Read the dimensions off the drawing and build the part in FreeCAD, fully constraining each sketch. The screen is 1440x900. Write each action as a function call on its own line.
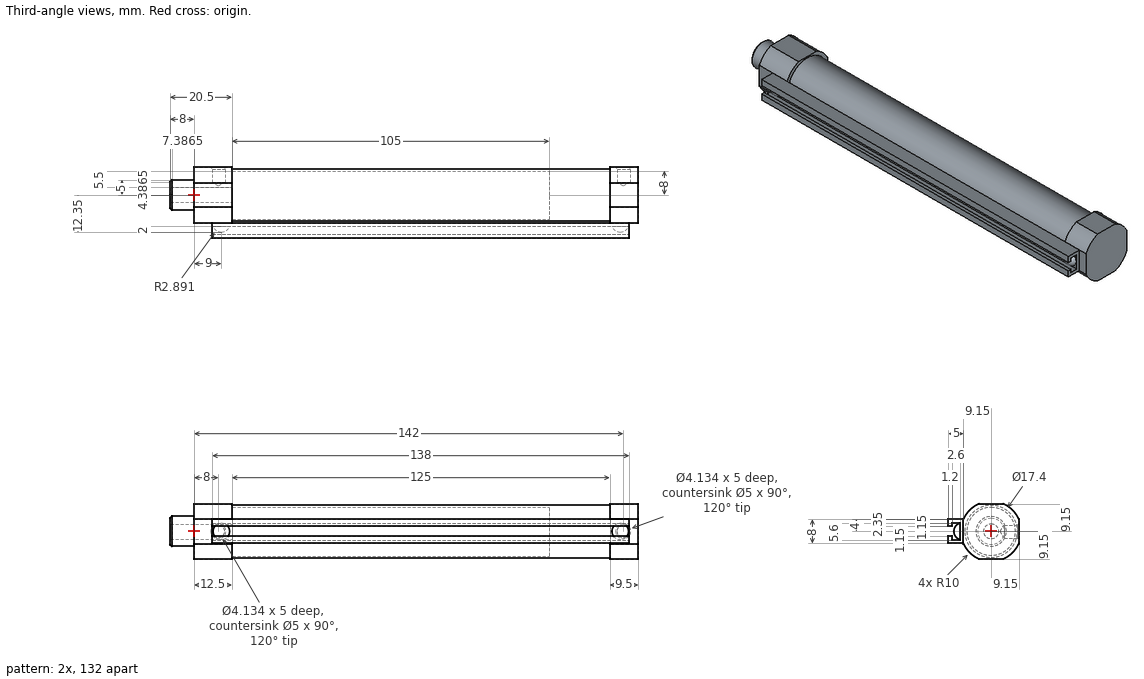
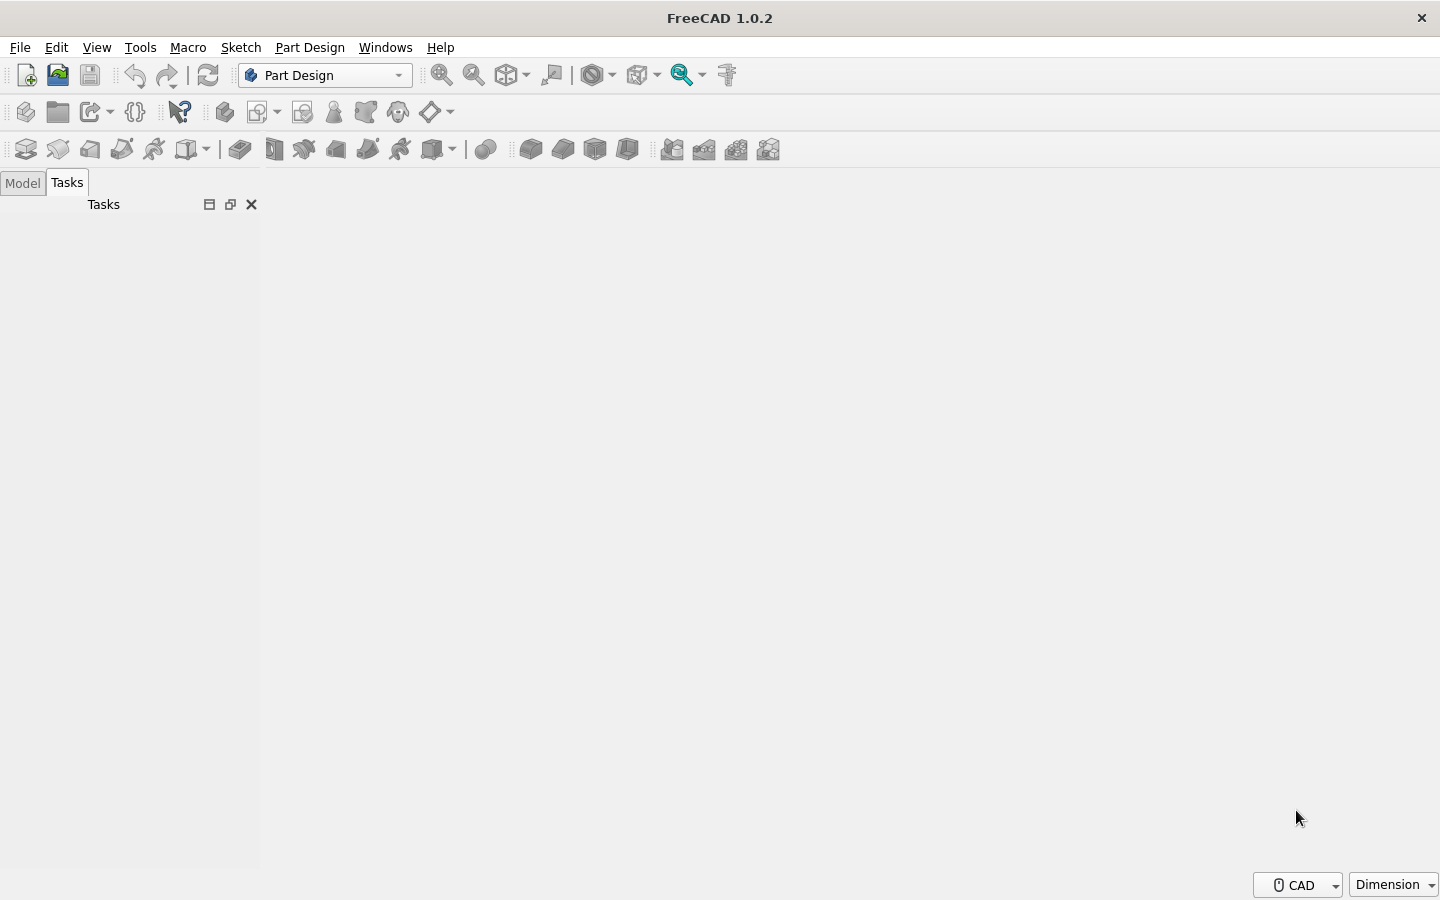
click(26, 76)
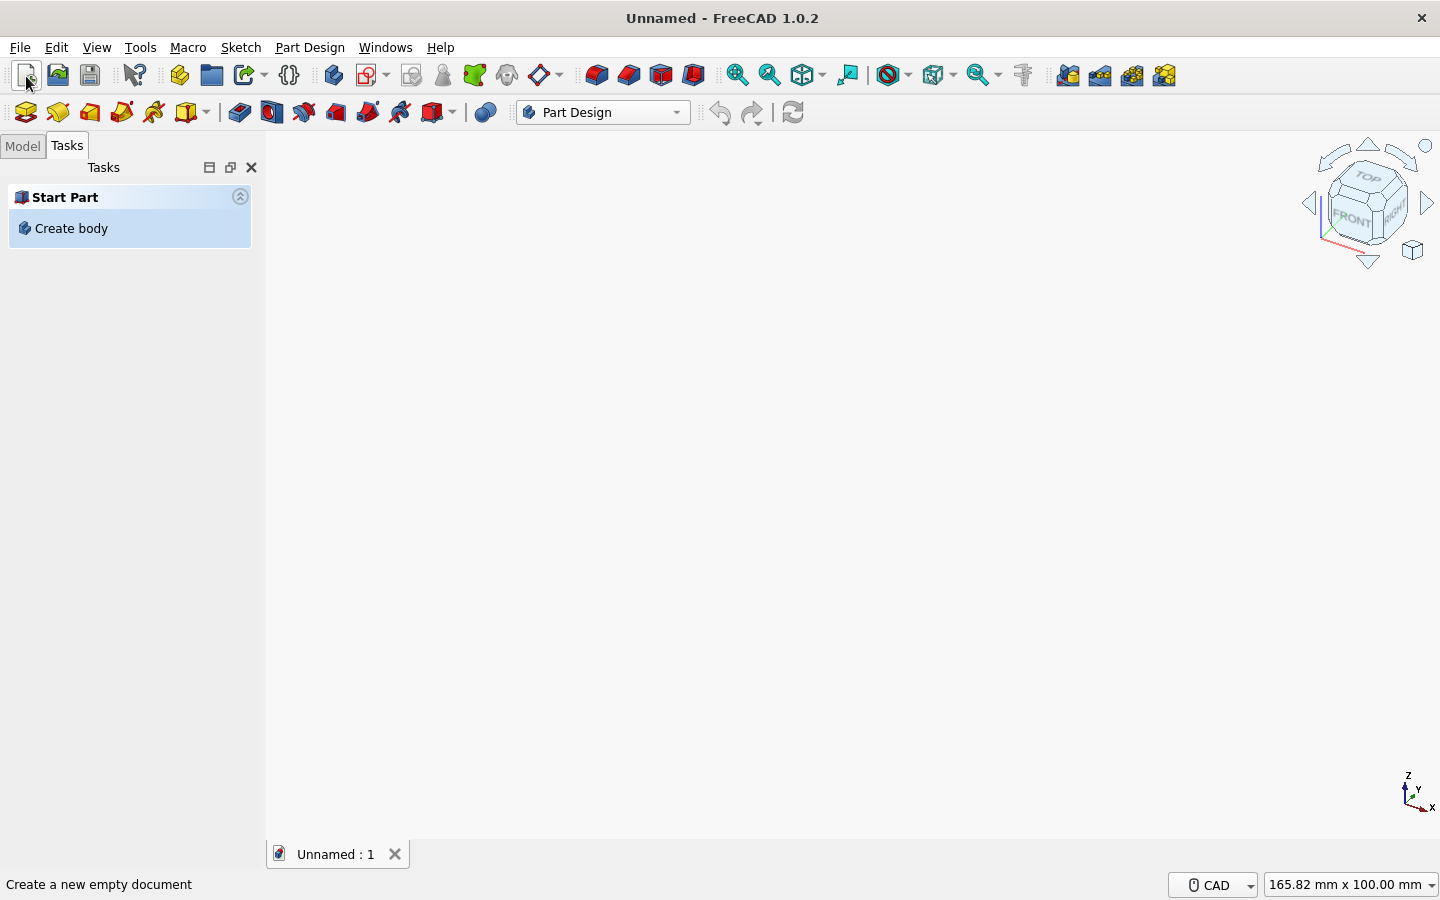
click(366, 76)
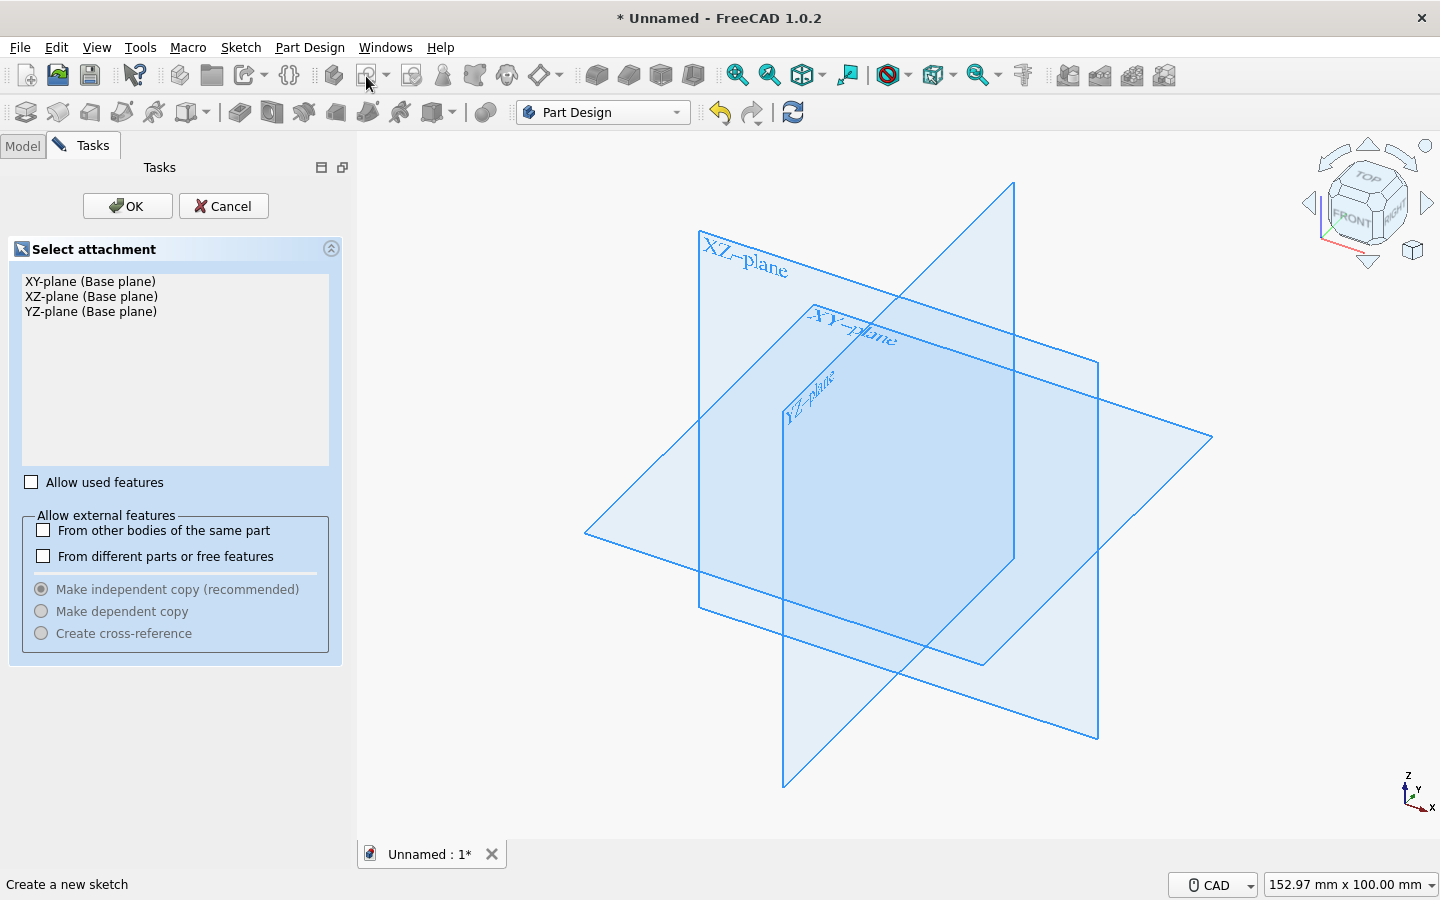
click(82, 282)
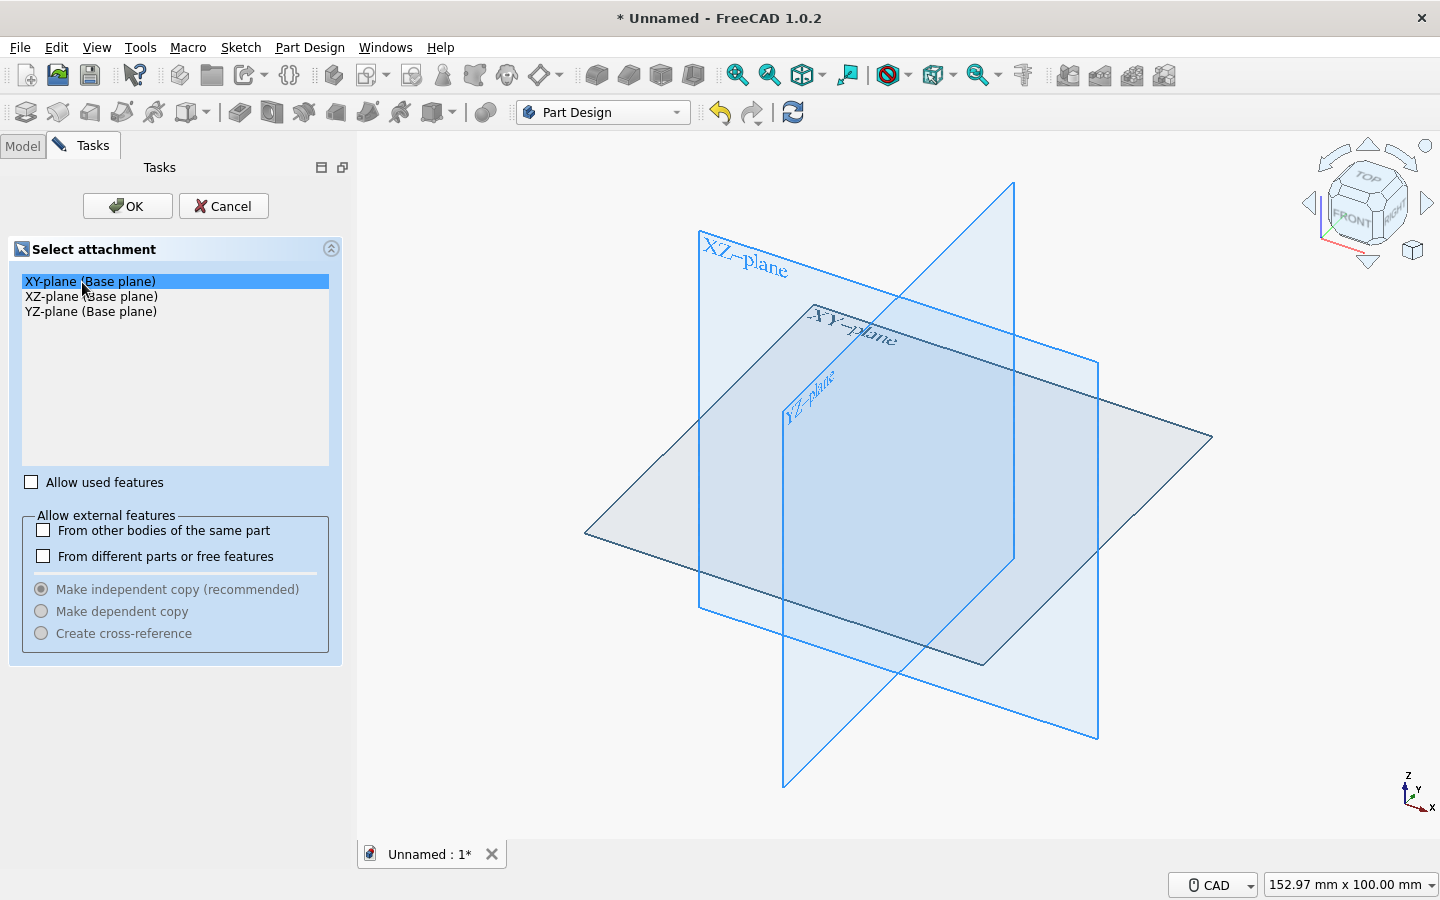
click(128, 206)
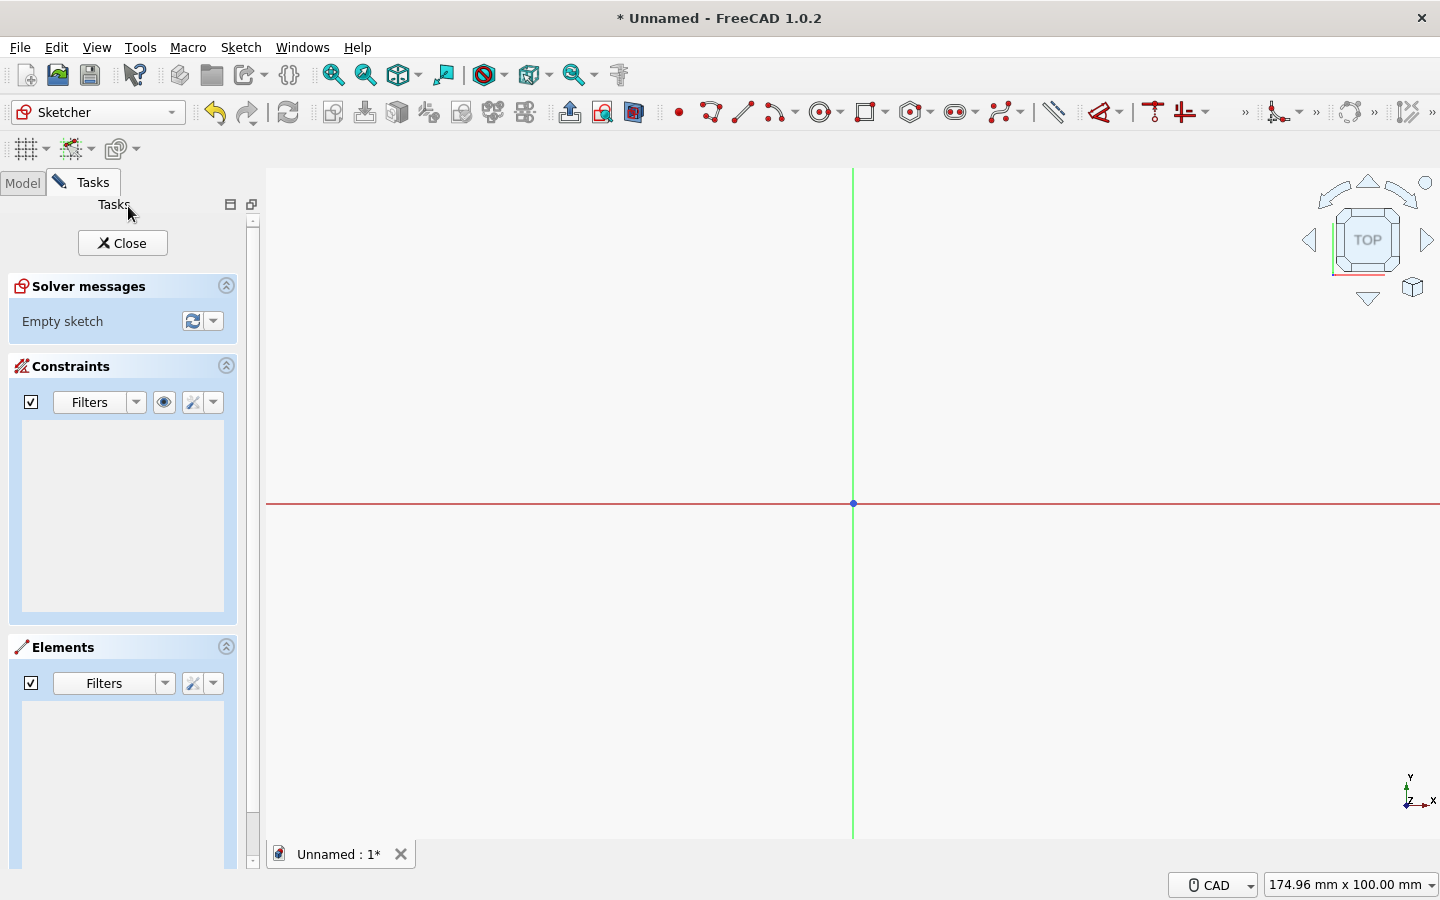
scroll(830, 485, up, 13)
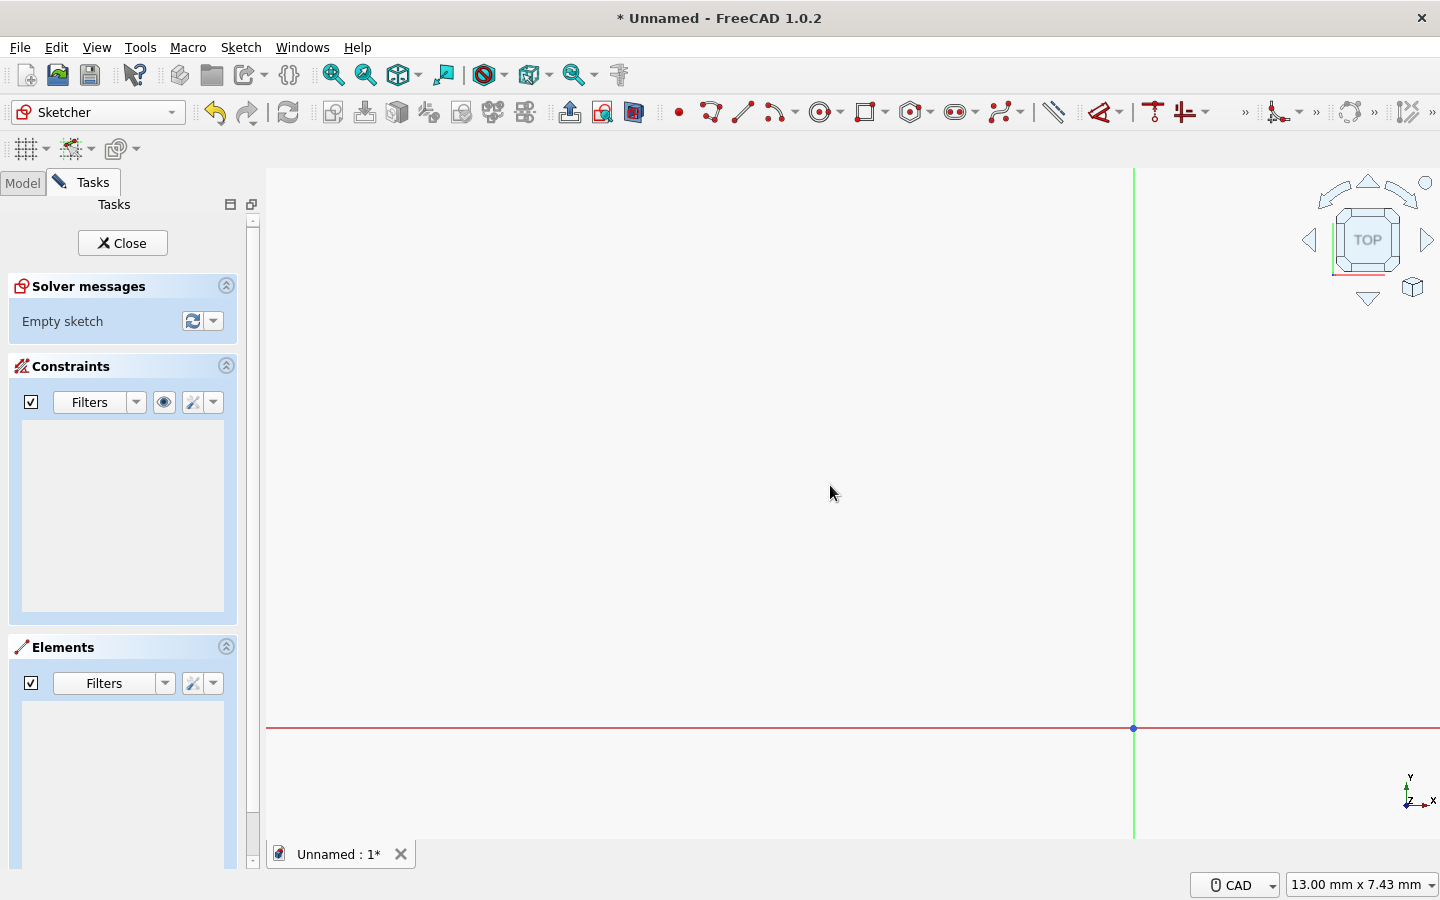
click(712, 112)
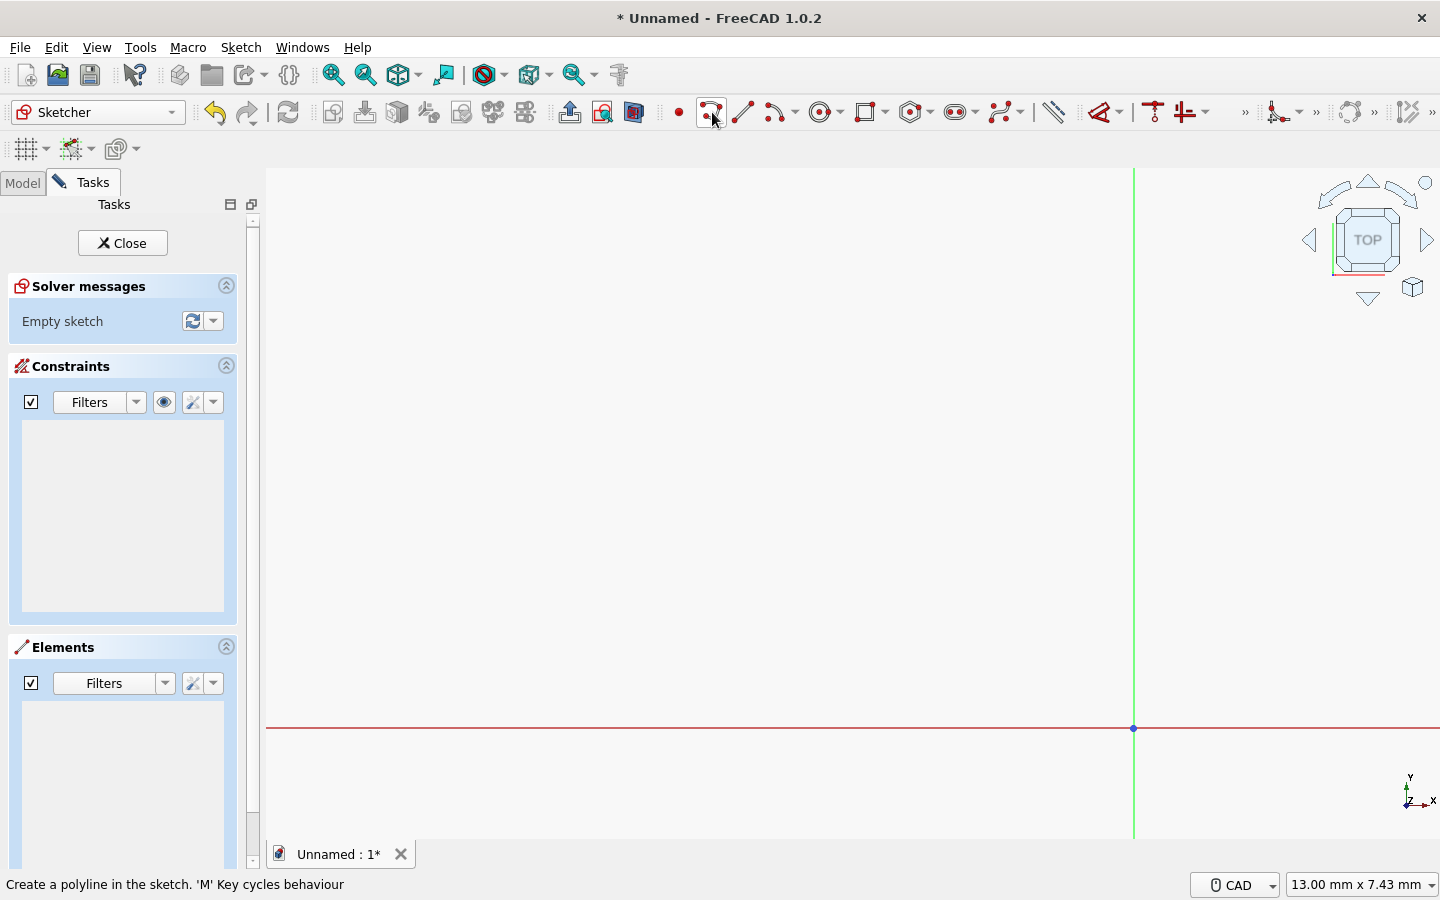
click(1134, 728)
click(1125, 276)
click(466, 276)
click(411, 332)
click(411, 719)
click(1134, 728)
key(Escape)
key(Escape)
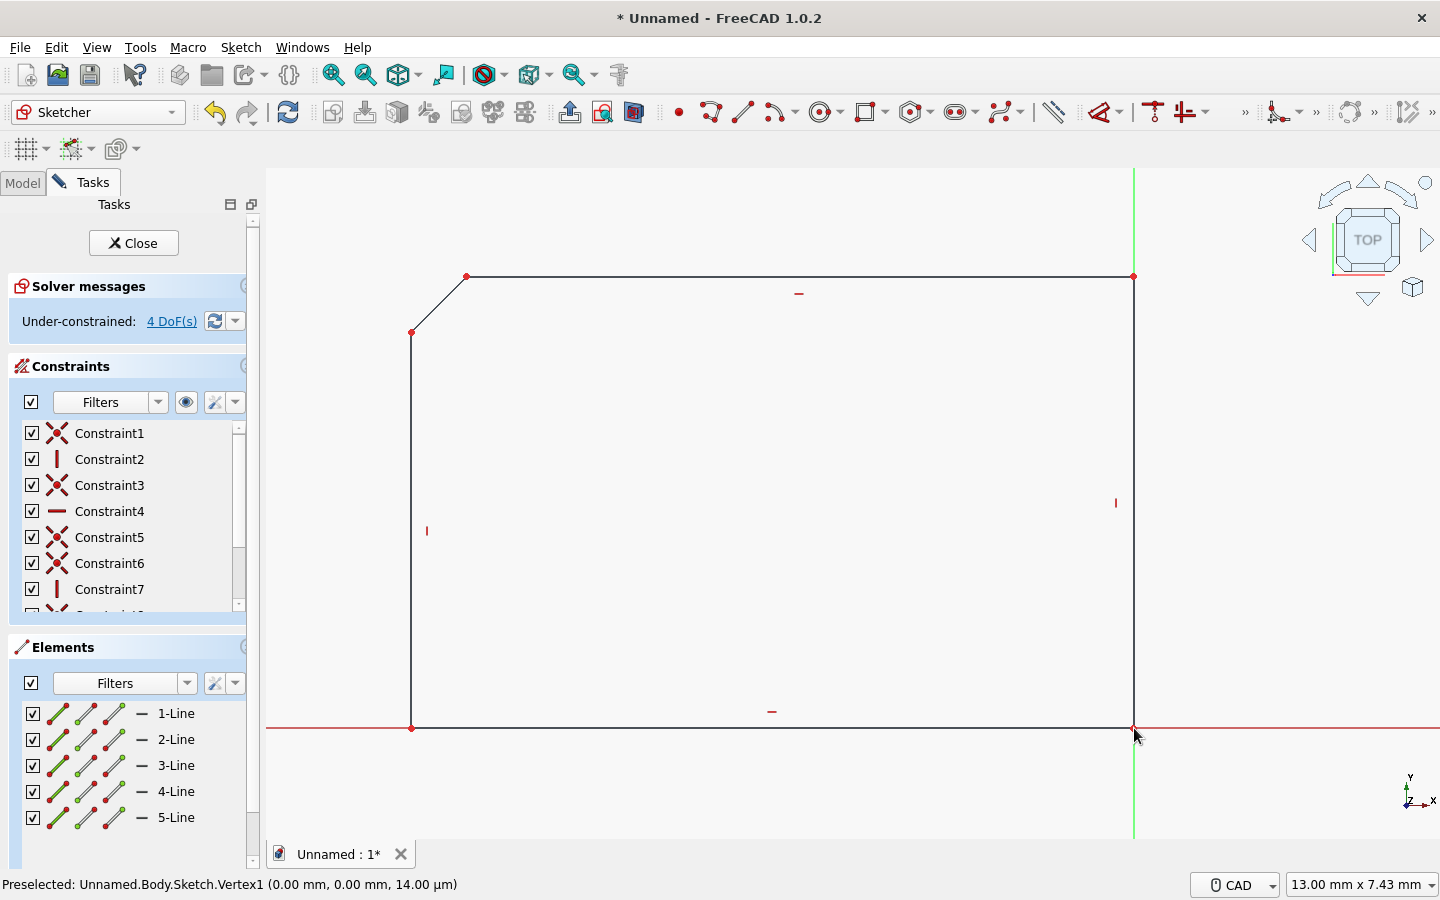
click(1100, 112)